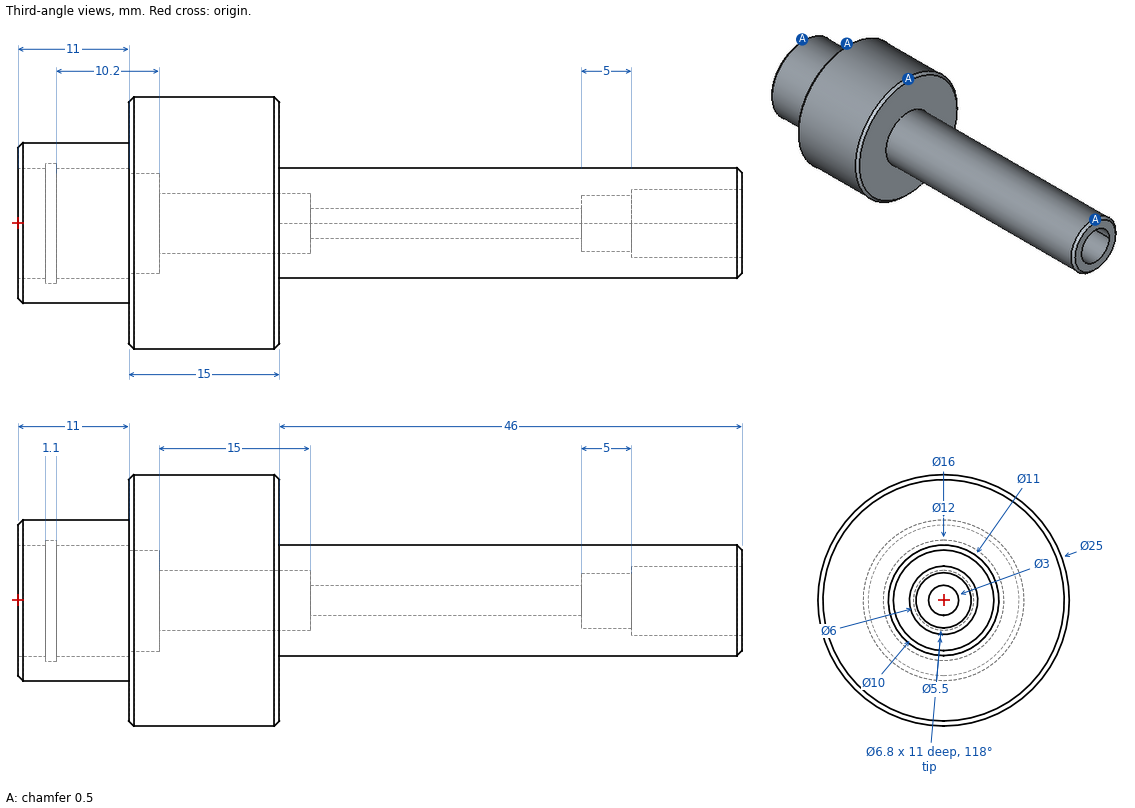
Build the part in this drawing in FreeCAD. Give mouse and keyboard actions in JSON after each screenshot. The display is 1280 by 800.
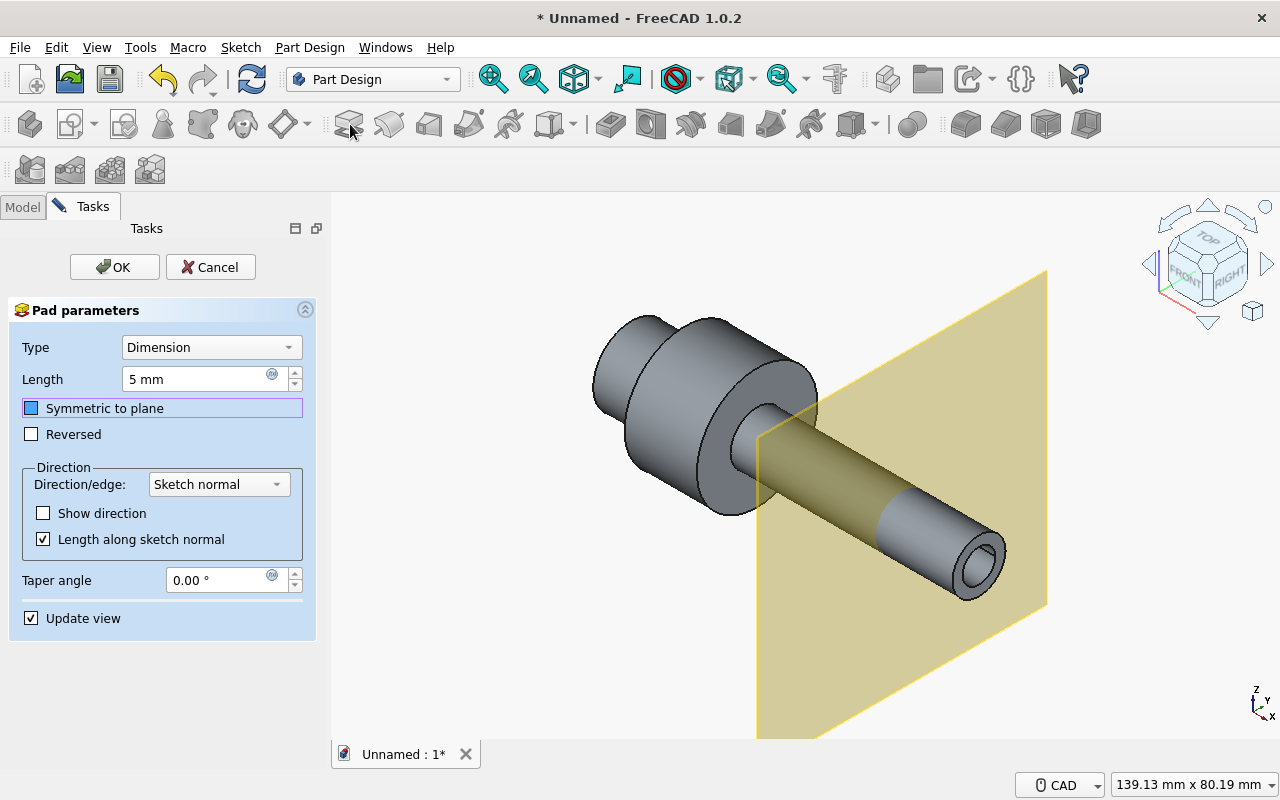
{"action": "left_click", "coordinate": [115, 267]}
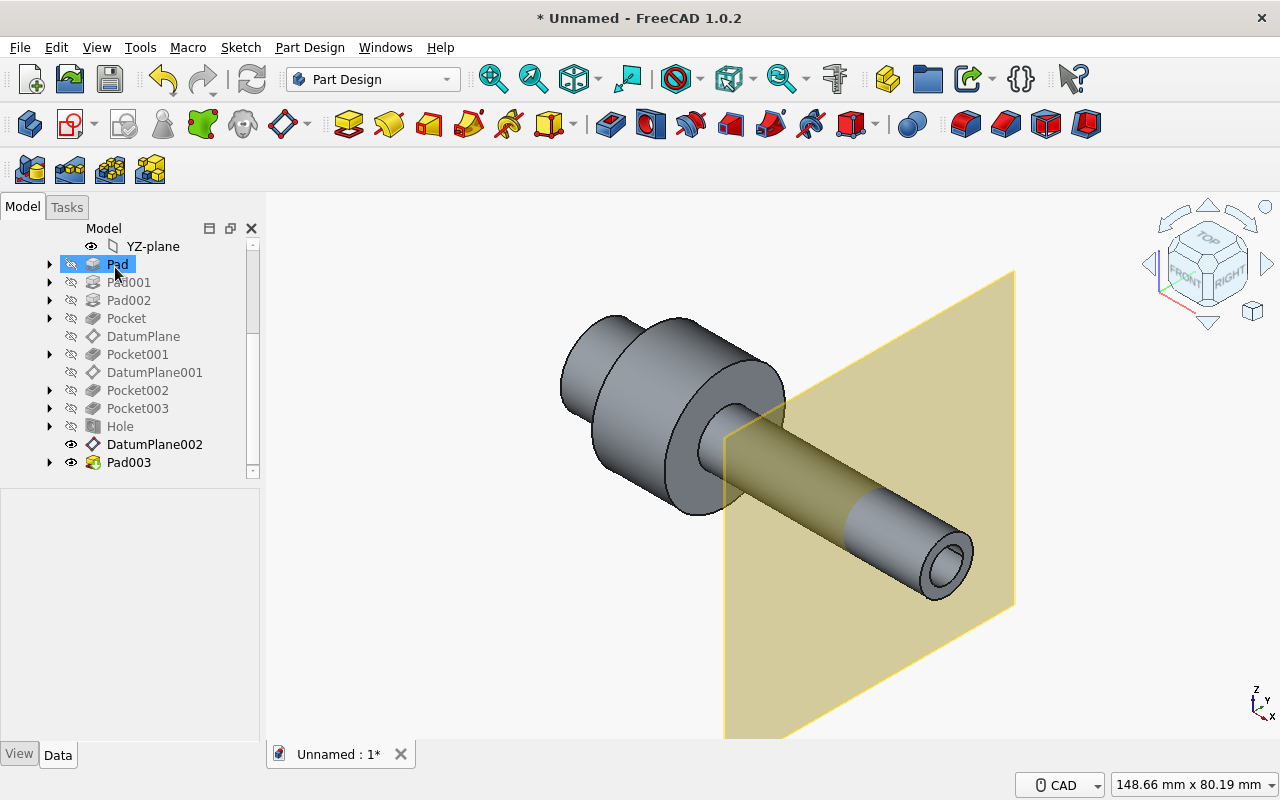
{"action": "left_click", "coordinate": [116, 444]}
{"action": "key", "text": "space"}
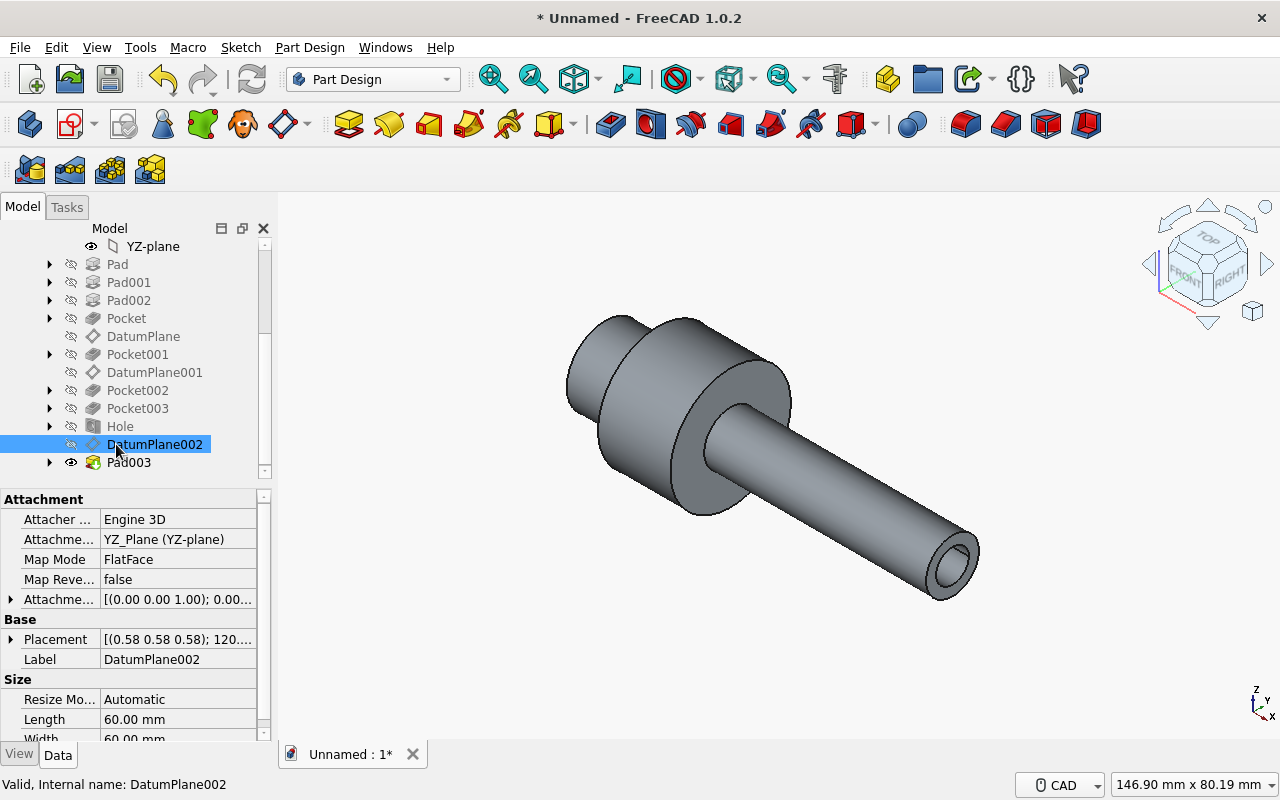
{"action": "key", "text": "3"}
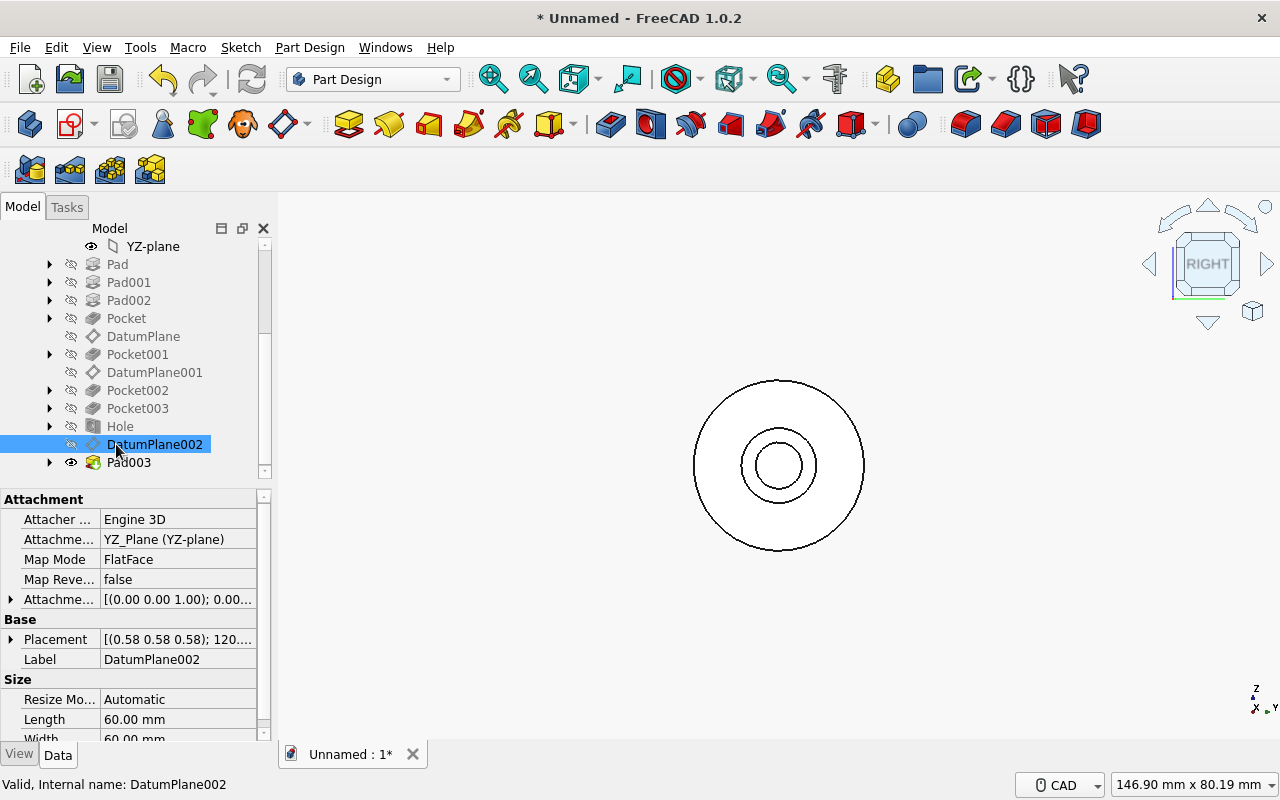
{"action": "left_click", "coordinate": [494, 80]}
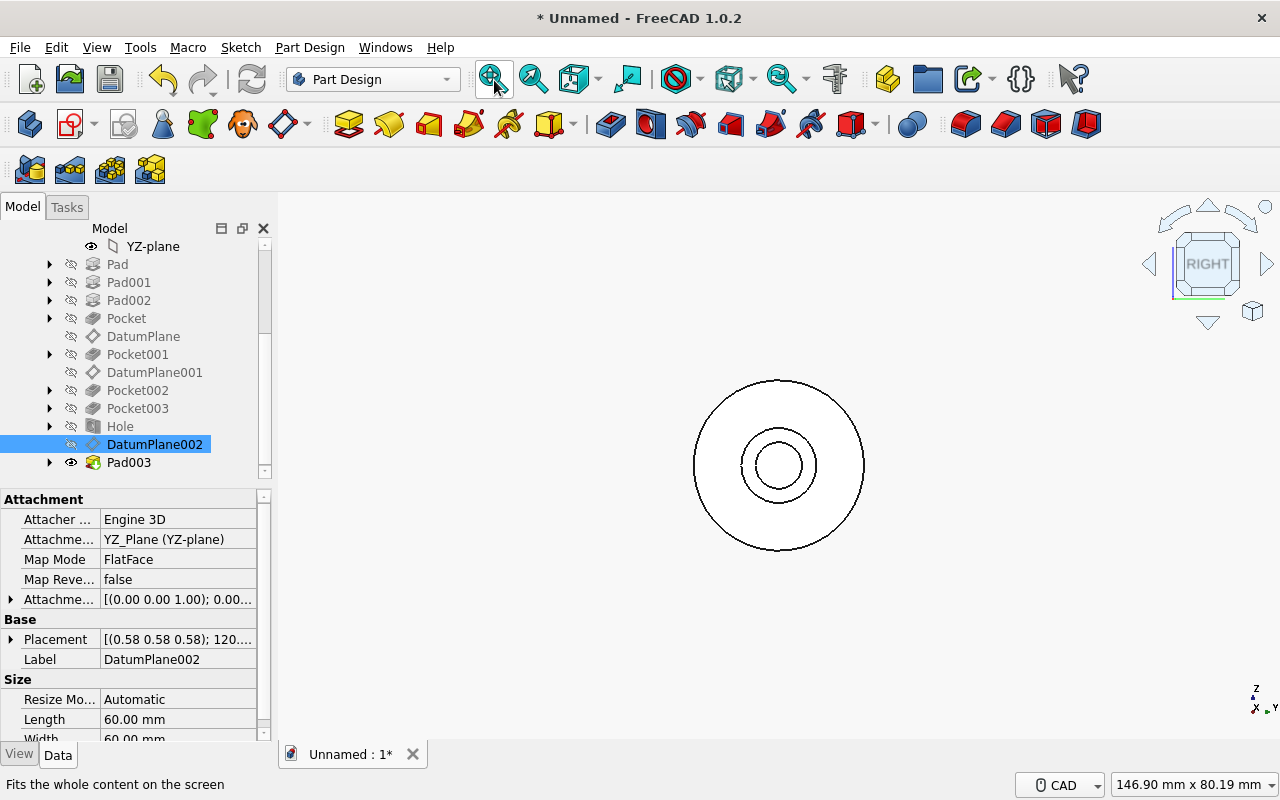
{"action": "left_click", "coordinate": [779, 464]}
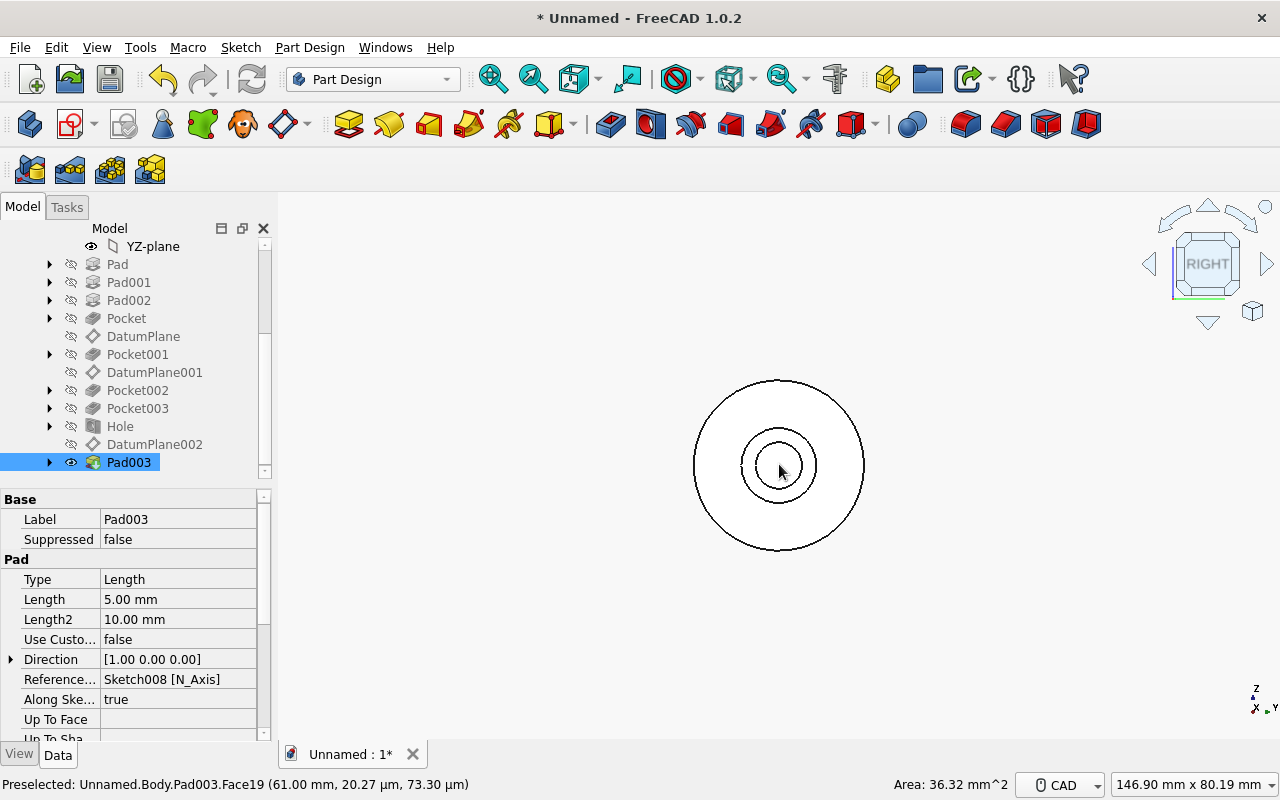
{"action": "left_click", "coordinate": [70, 124]}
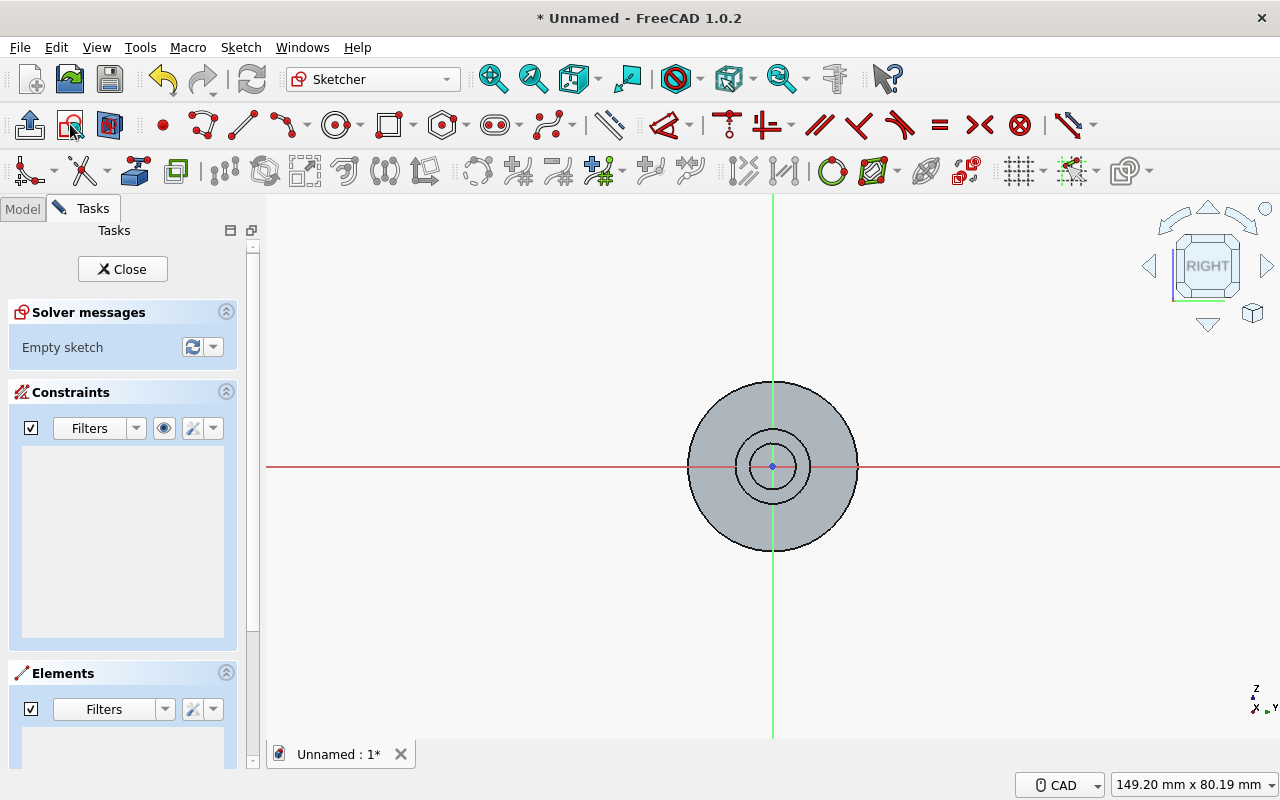
{"action": "key", "text": "q s"}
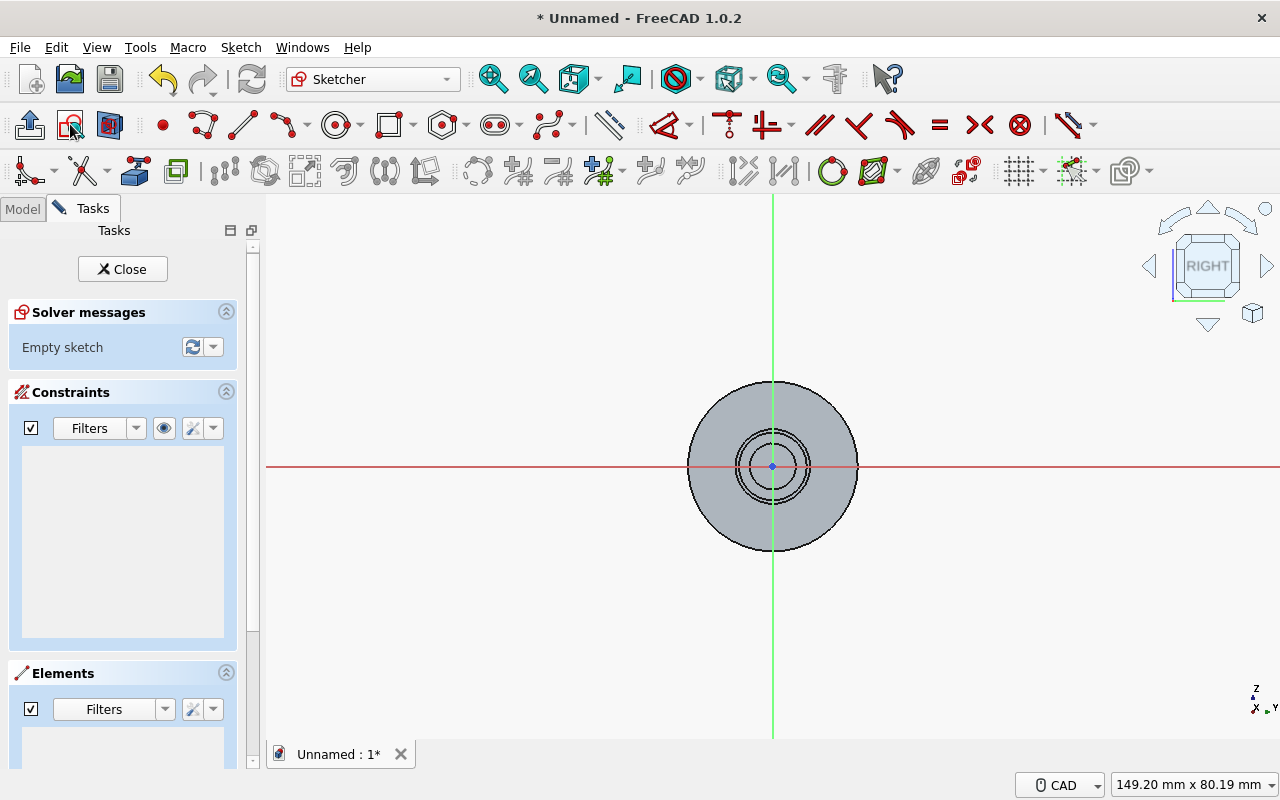
{"action": "scroll", "coordinate": [781, 466], "scroll_direction": "up", "scroll_amount": 11}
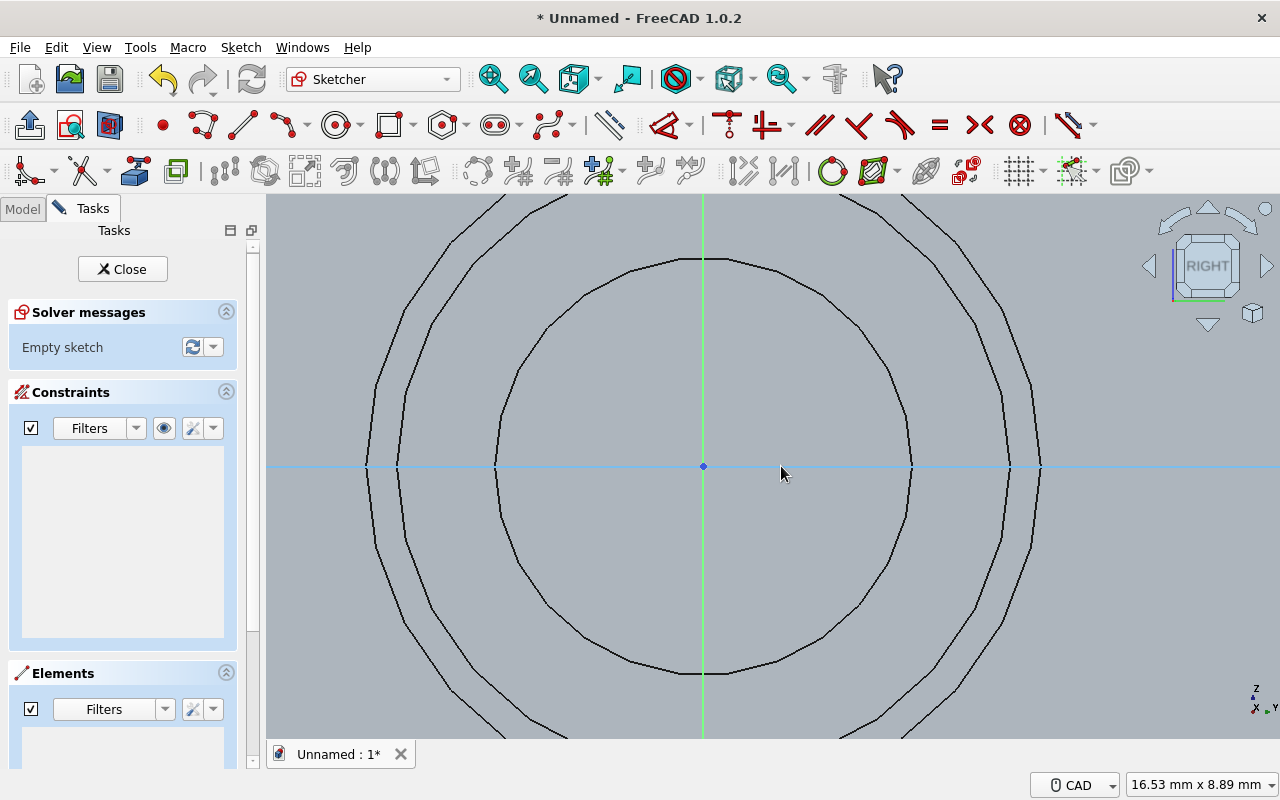
{"action": "left_click", "coordinate": [336, 126]}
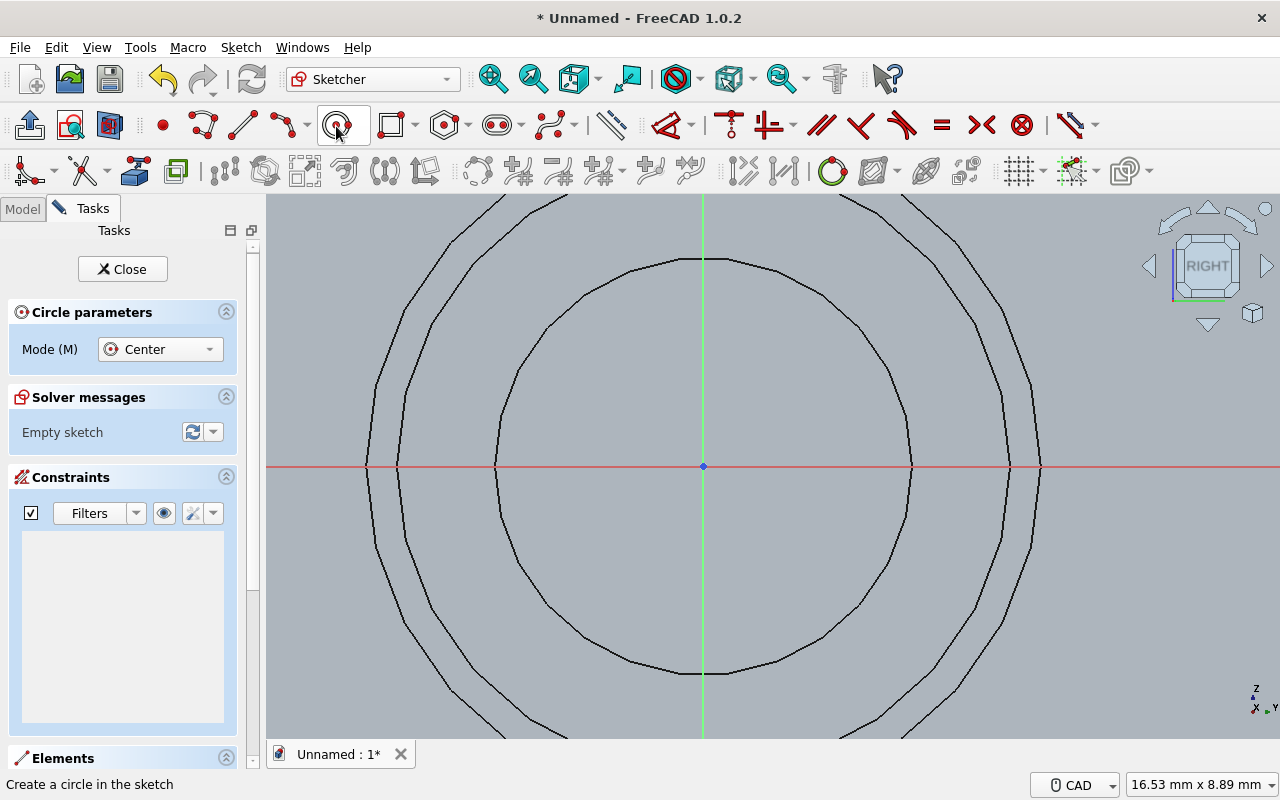
{"action": "left_click", "coordinate": [703, 466]}
{"action": "mouse_move", "coordinate": [823, 347]}